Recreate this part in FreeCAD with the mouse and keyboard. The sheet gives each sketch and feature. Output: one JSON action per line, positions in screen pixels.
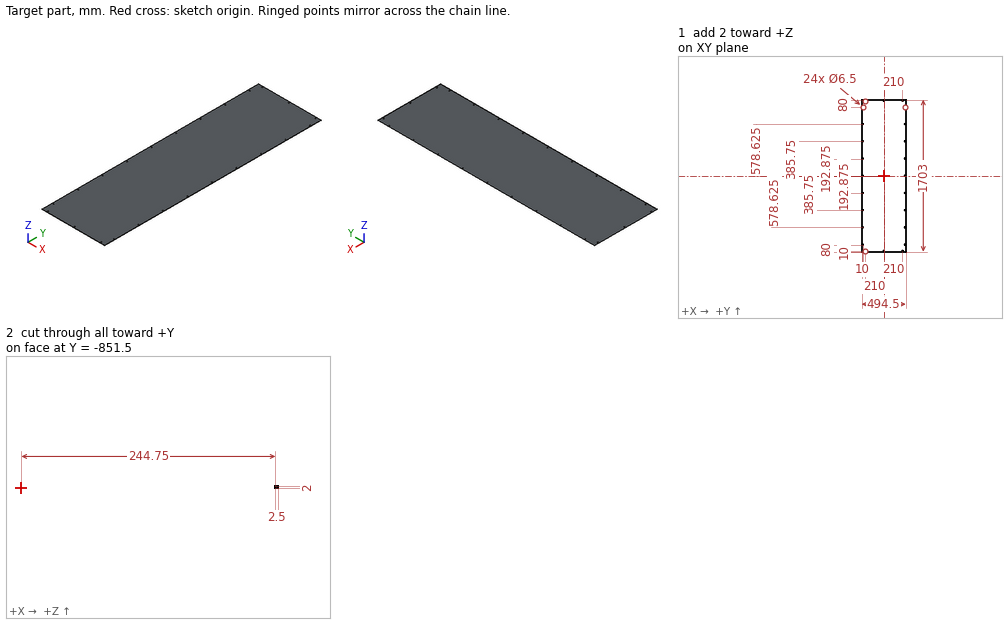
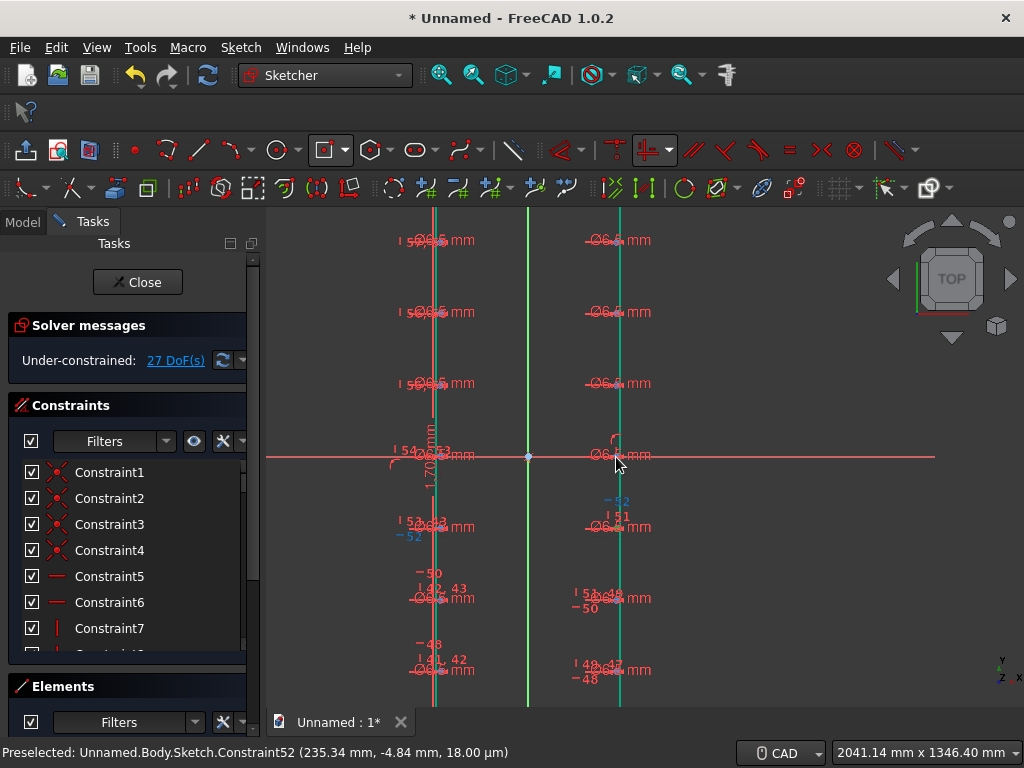
{"action": "left_click", "coordinate": [616, 457]}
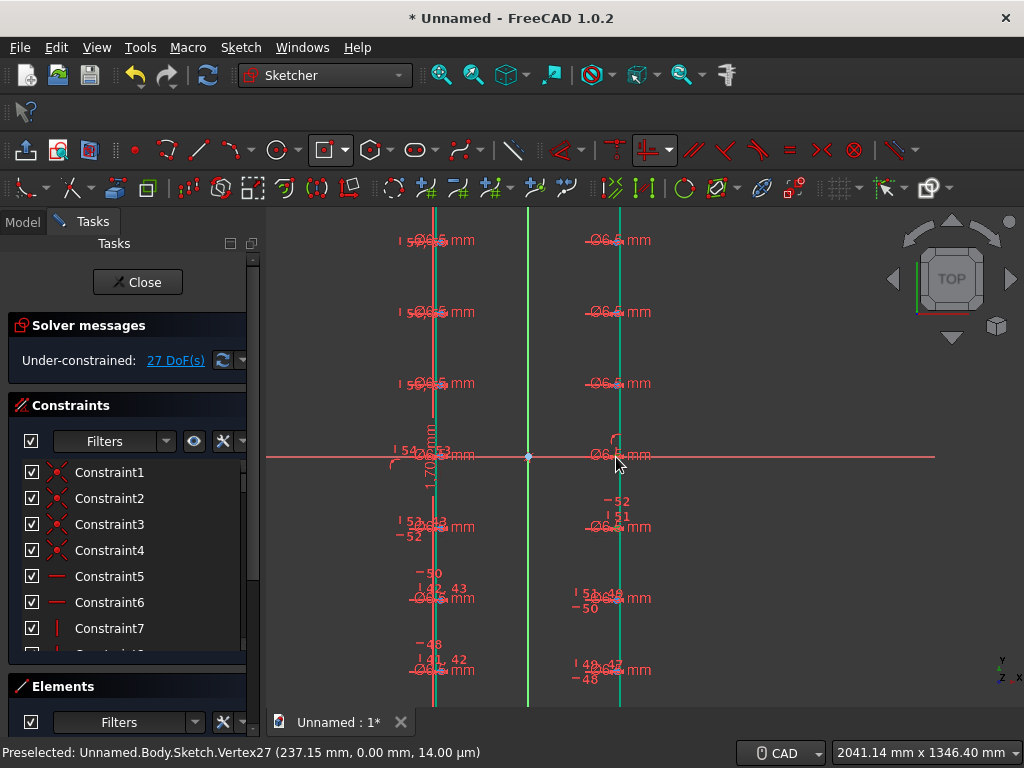
{"action": "key", "text": "v"}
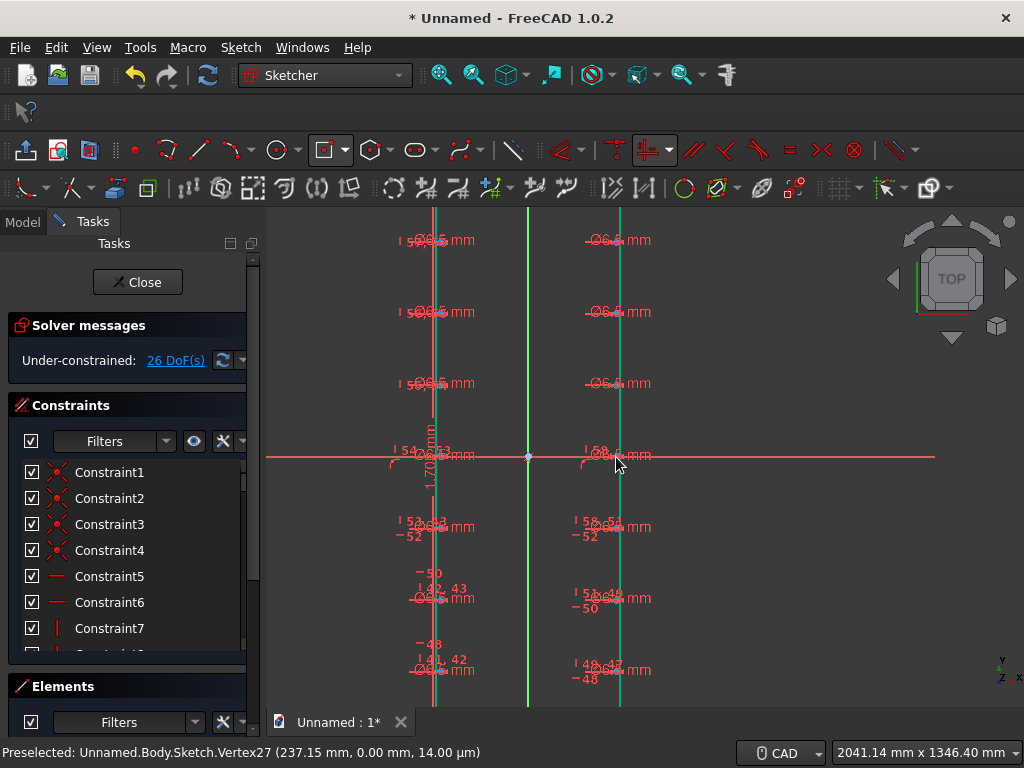
{"action": "left_click", "coordinate": [616, 457]}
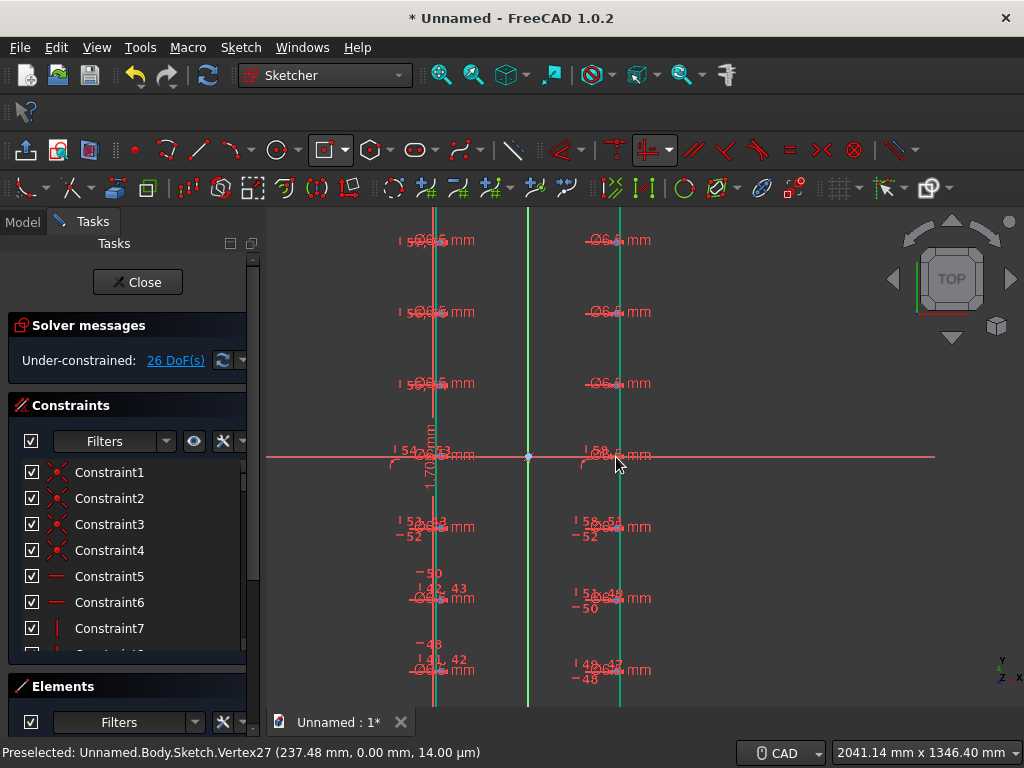
{"action": "left_click", "coordinate": [616, 385]}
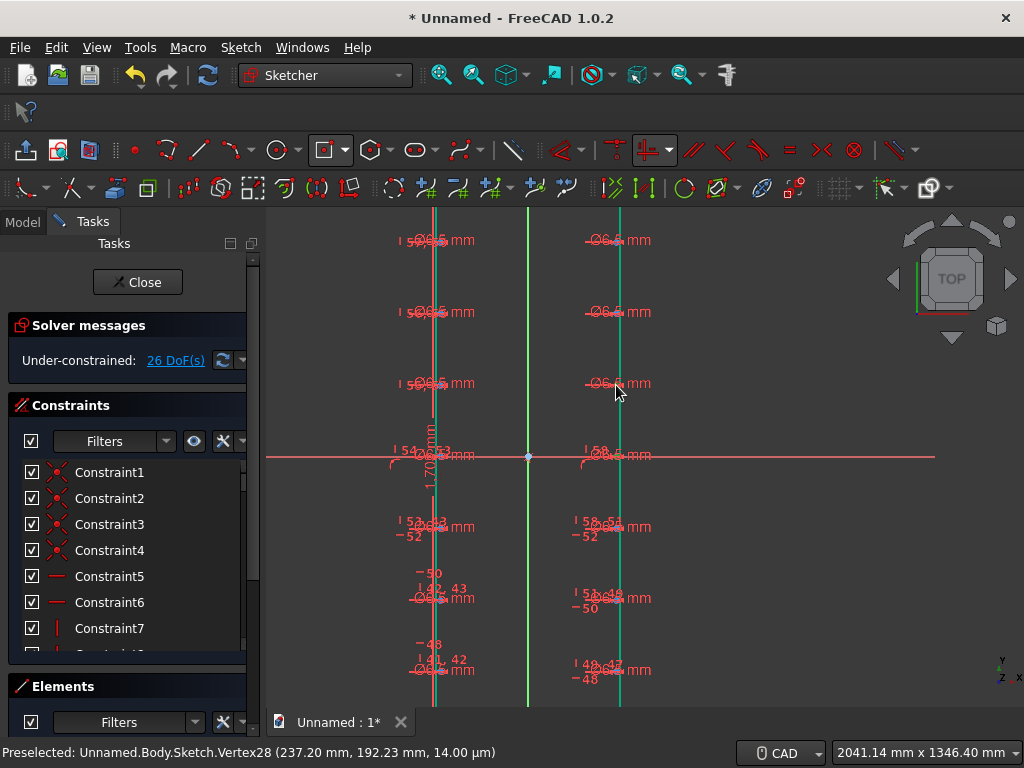
{"action": "key", "text": "v"}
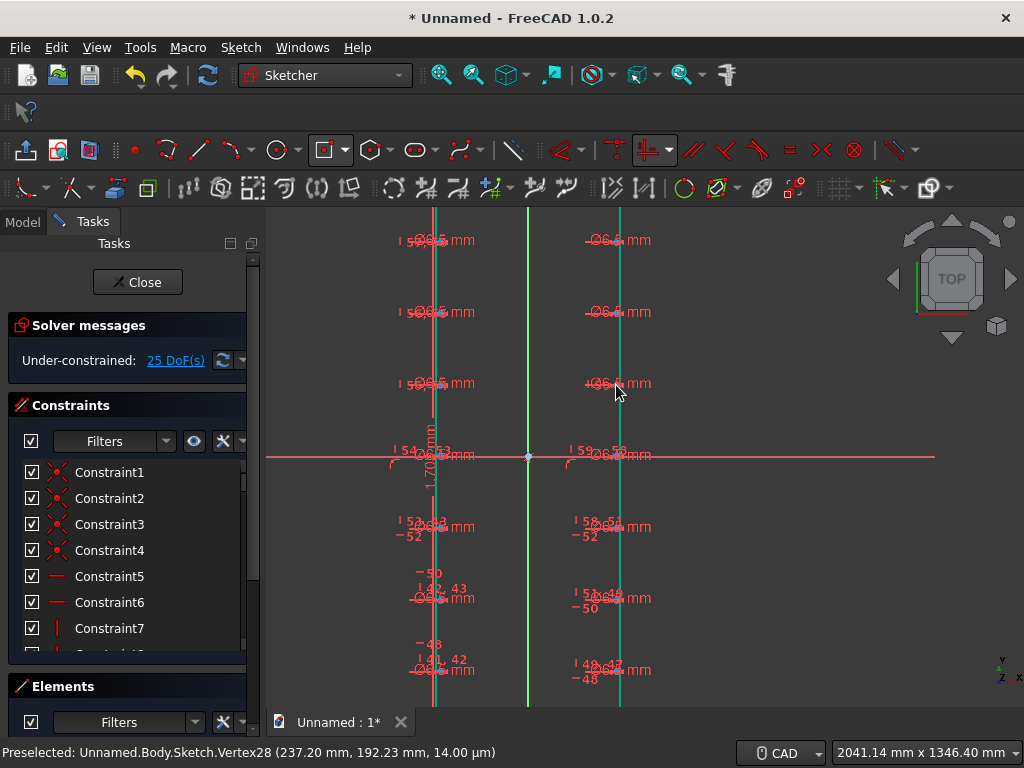
{"action": "left_click", "coordinate": [440, 385]}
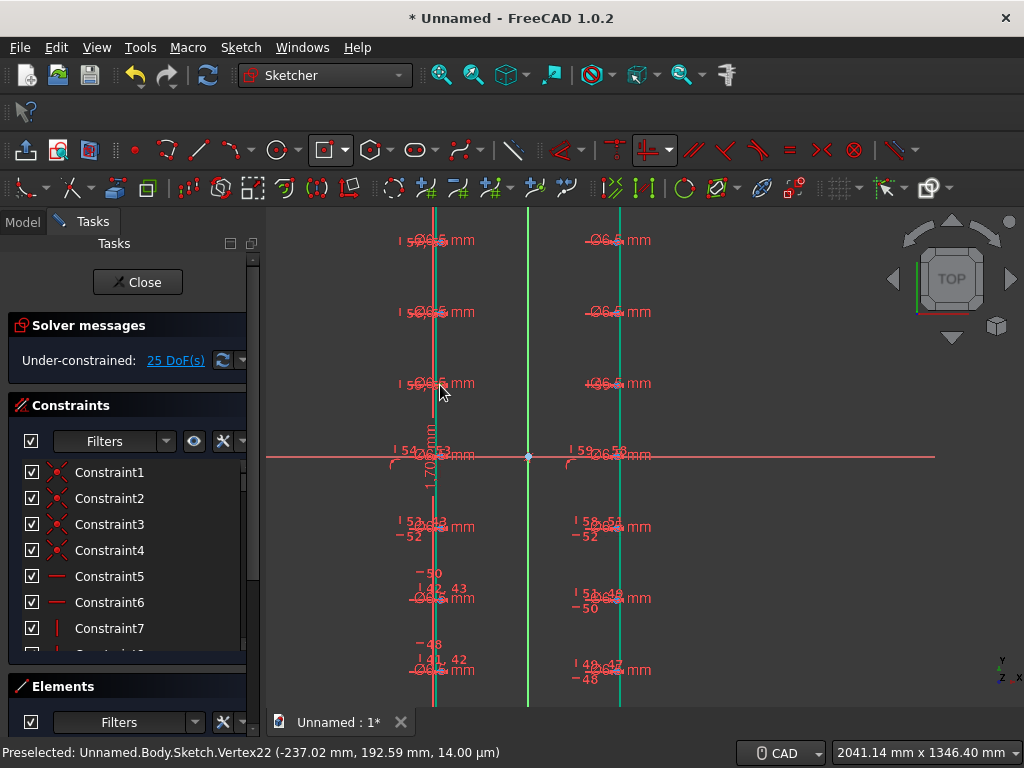
{"action": "left_click", "coordinate": [616, 385]}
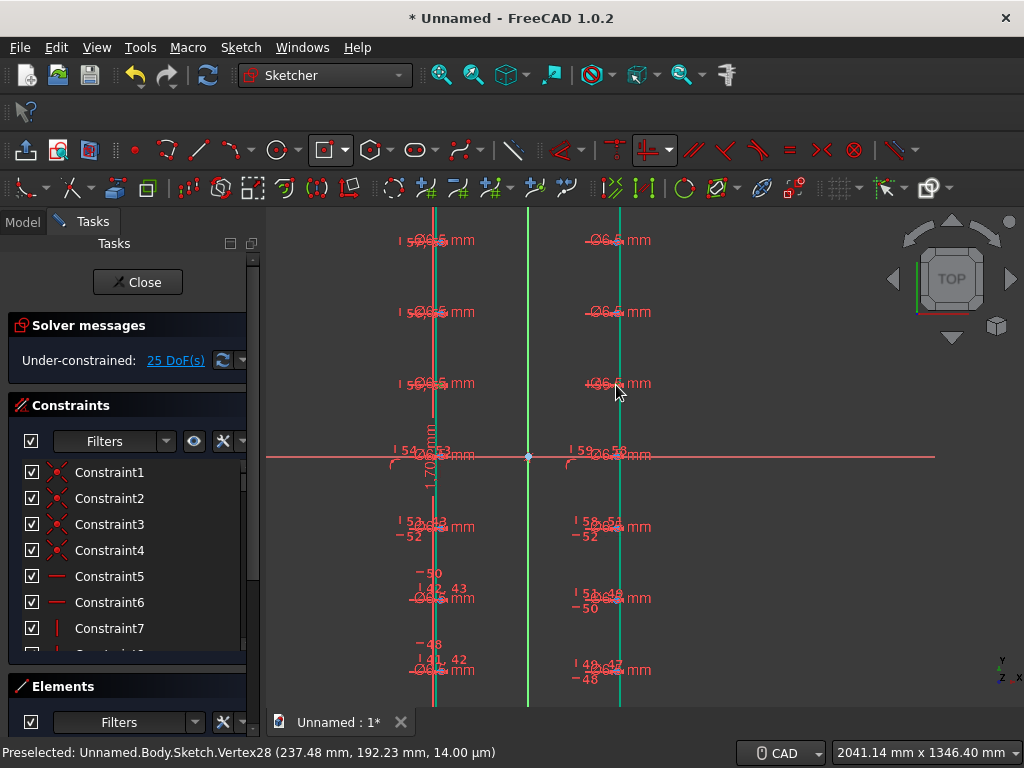
{"action": "left_click", "coordinate": [672, 150]}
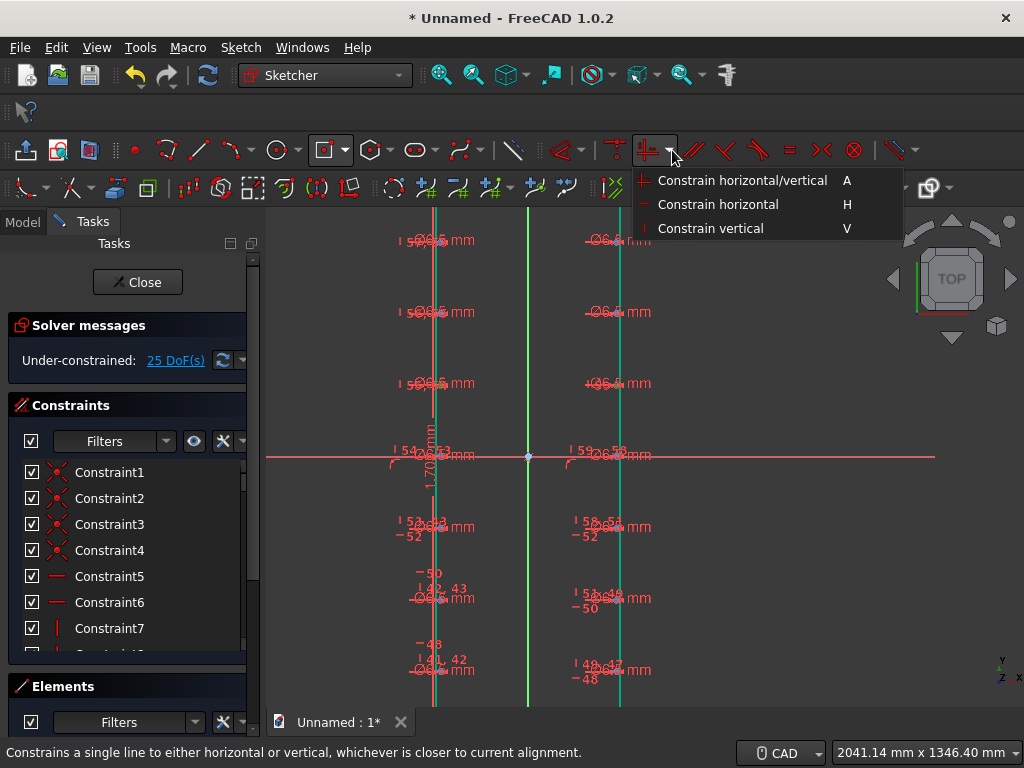
{"action": "left_click", "coordinate": [768, 204]}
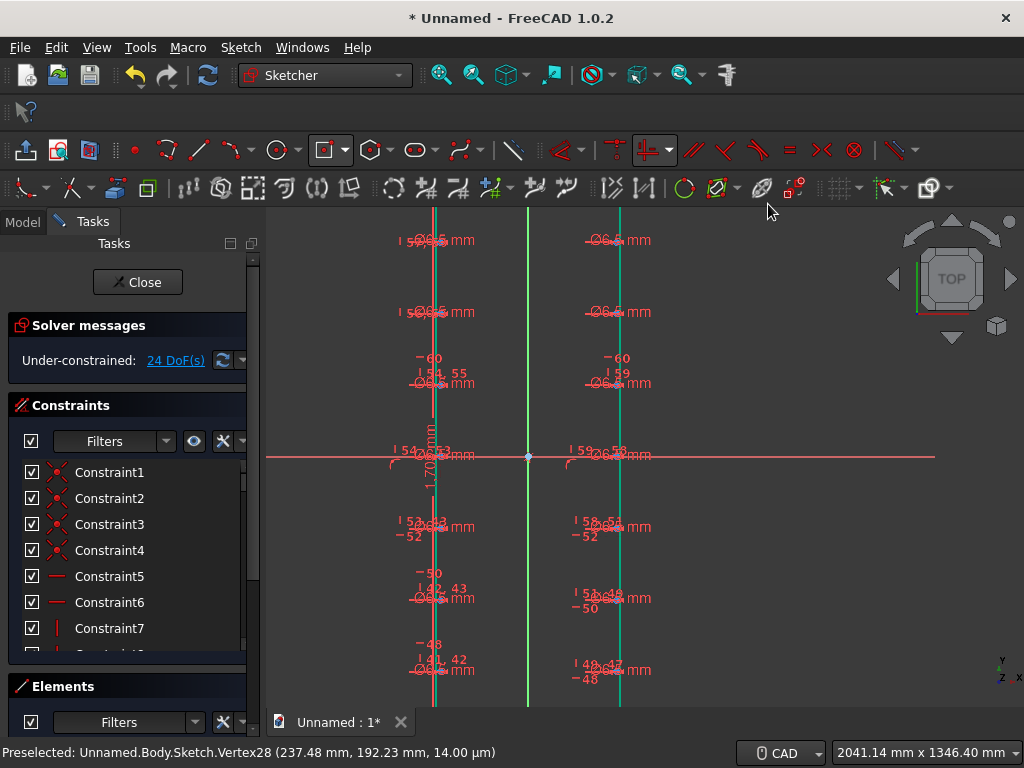
{"action": "left_click", "coordinate": [616, 385]}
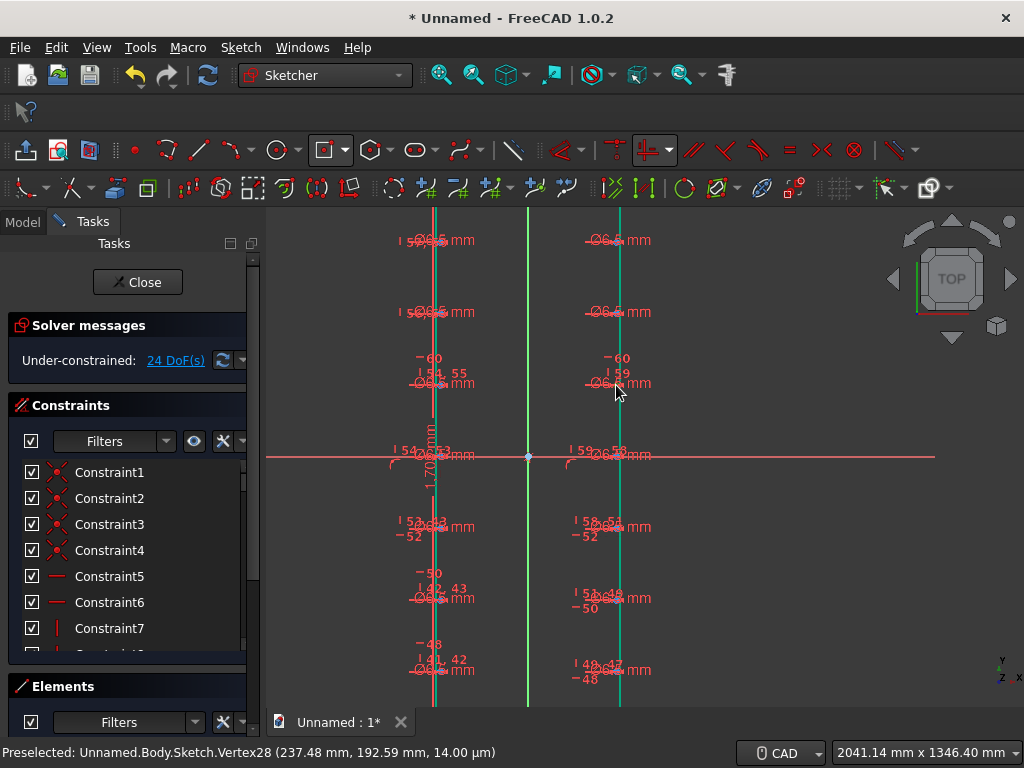
{"action": "left_click", "coordinate": [616, 314]}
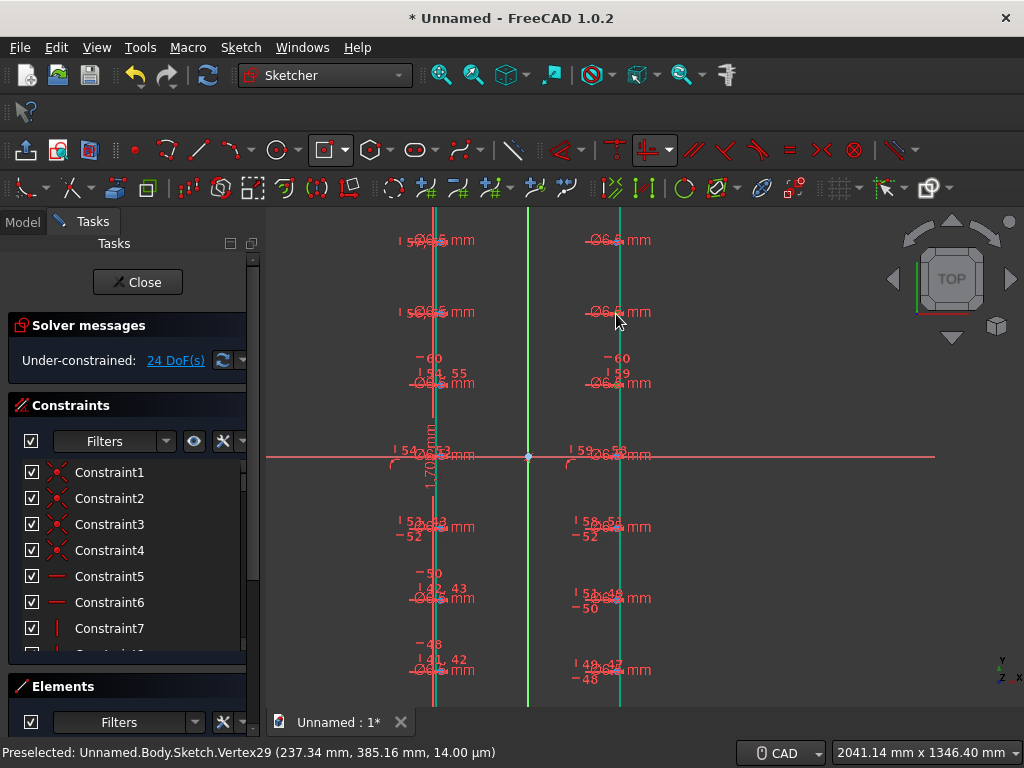
{"action": "left_click", "coordinate": [672, 150]}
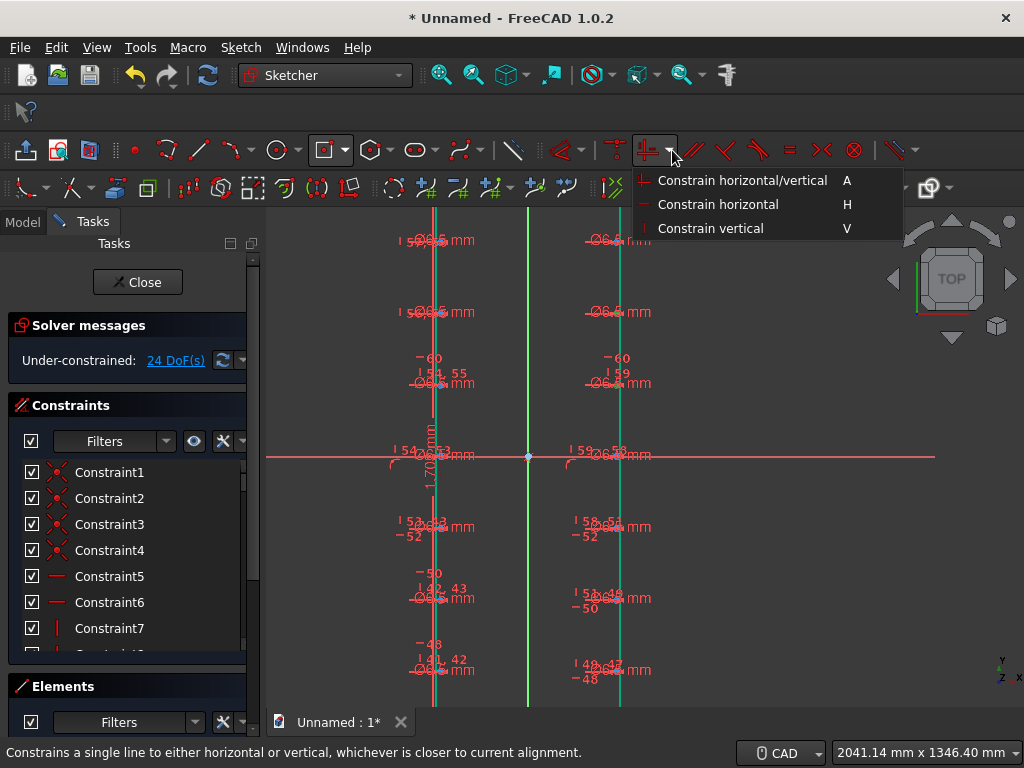
{"action": "left_click", "coordinate": [768, 228]}